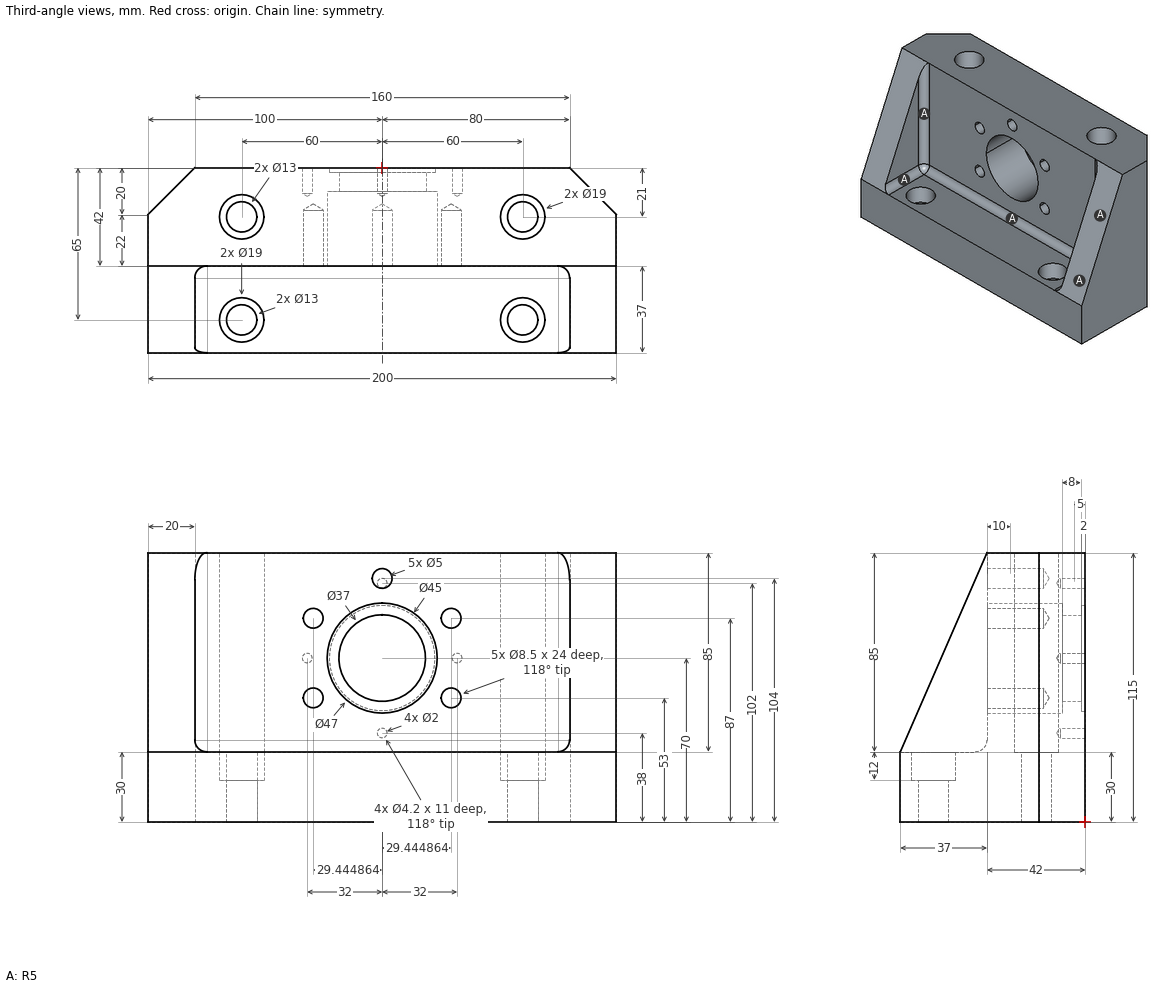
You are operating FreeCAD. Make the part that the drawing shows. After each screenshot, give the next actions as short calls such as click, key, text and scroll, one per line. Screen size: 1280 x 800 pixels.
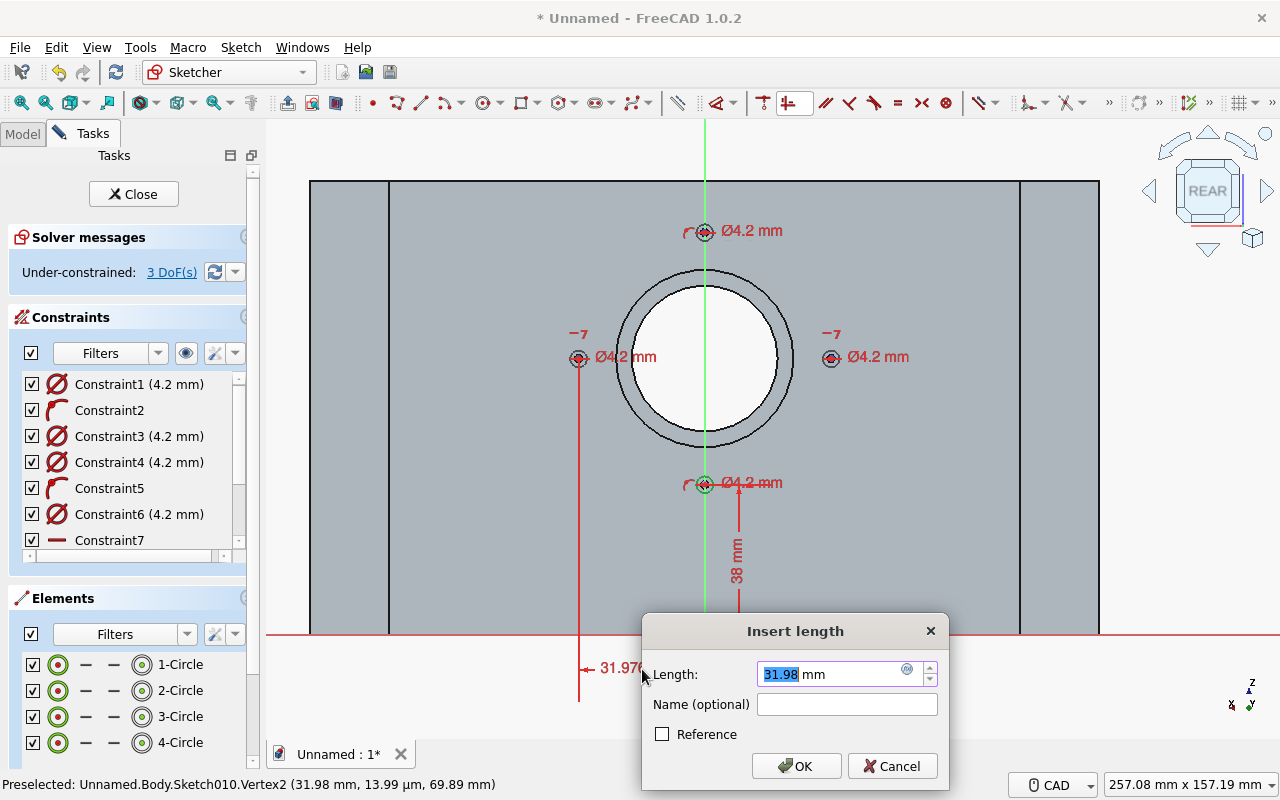
text(32)
key(Return)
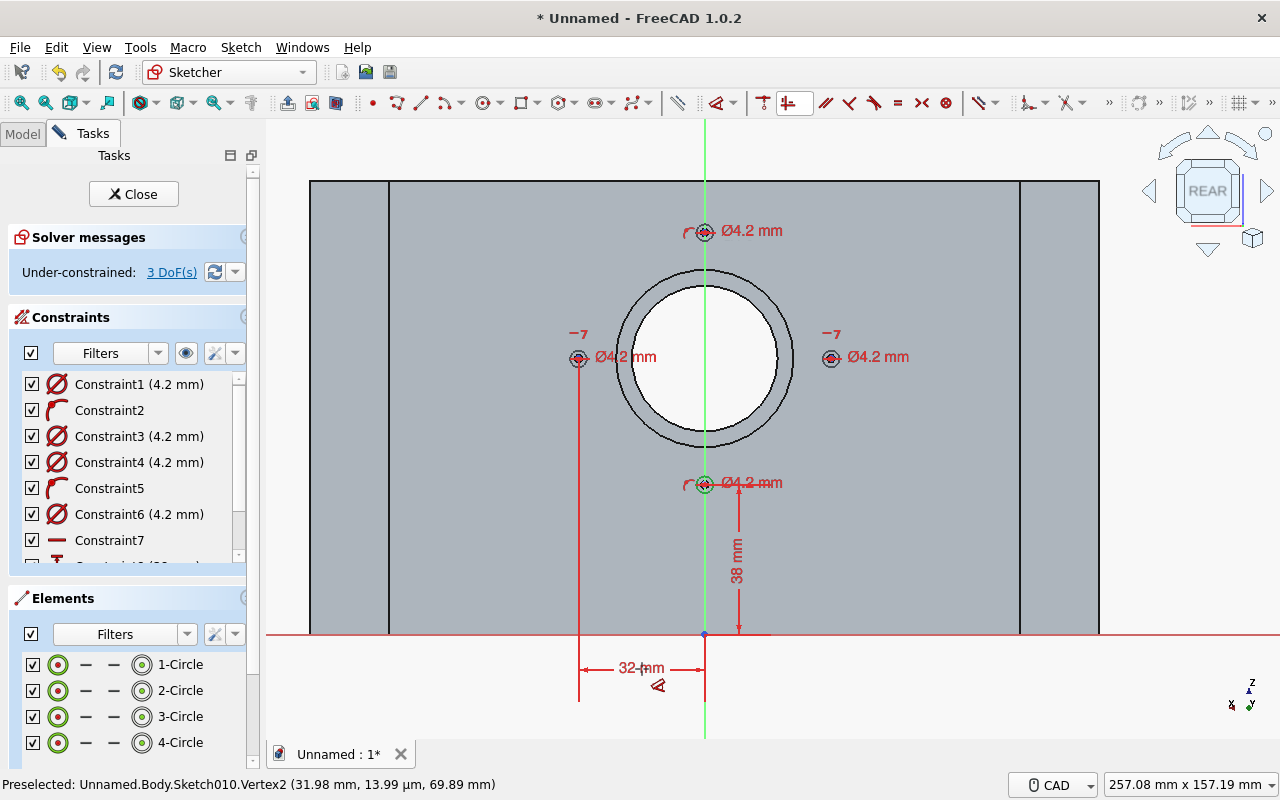
click(579, 359)
click(545, 497)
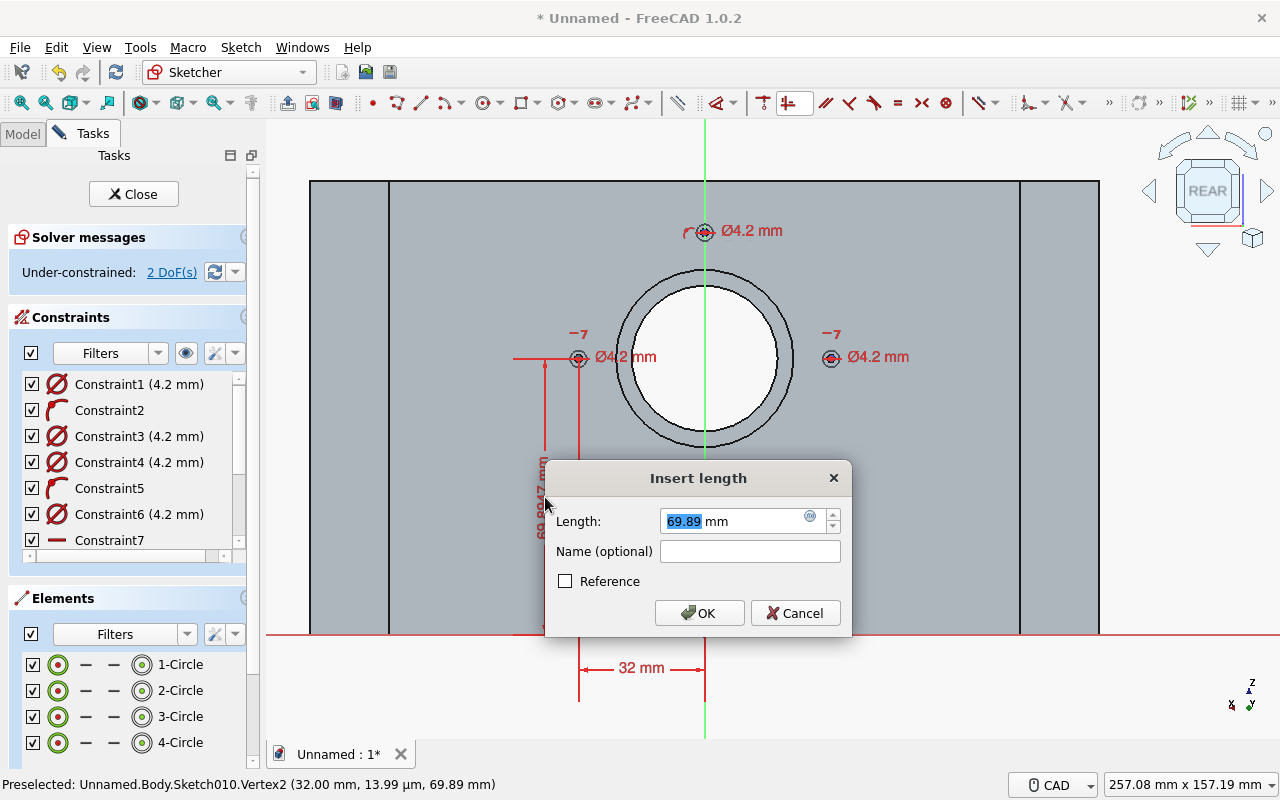
text(70)
key(Return)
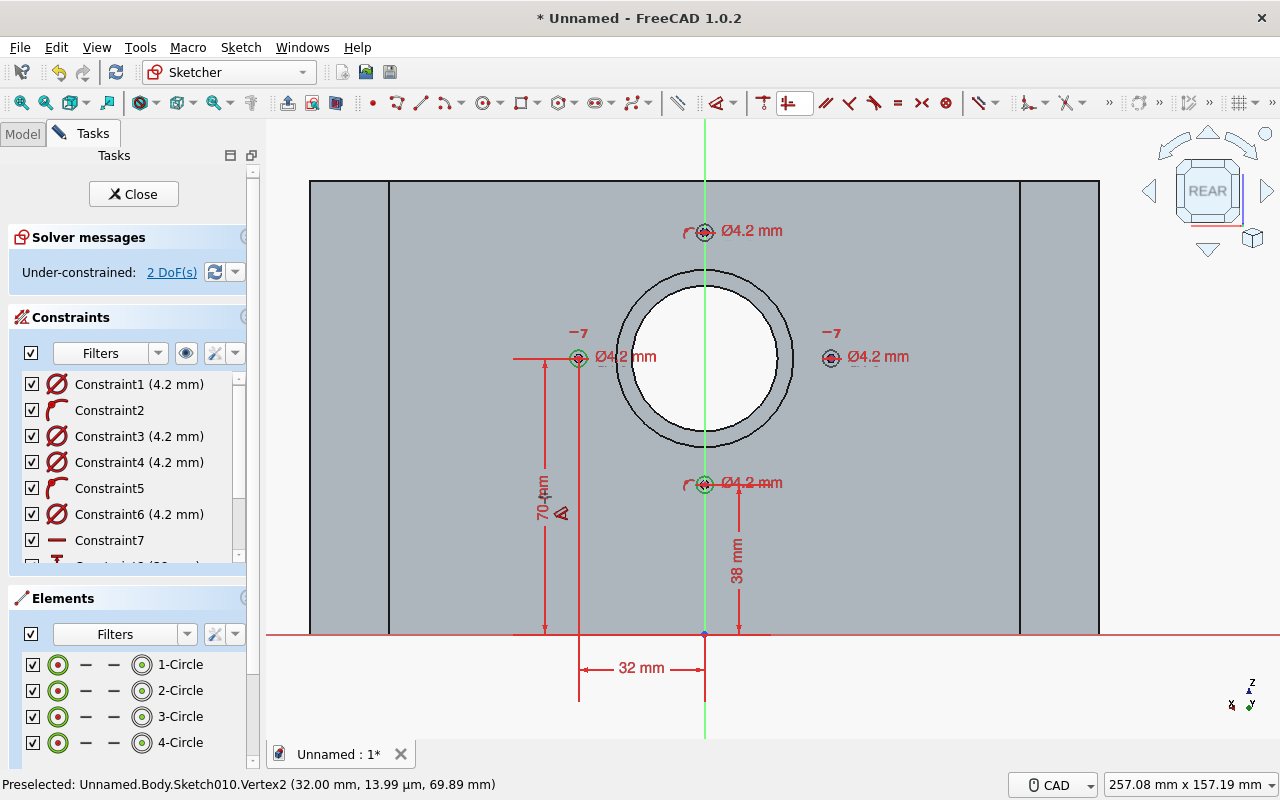
click(831, 359)
click(768, 669)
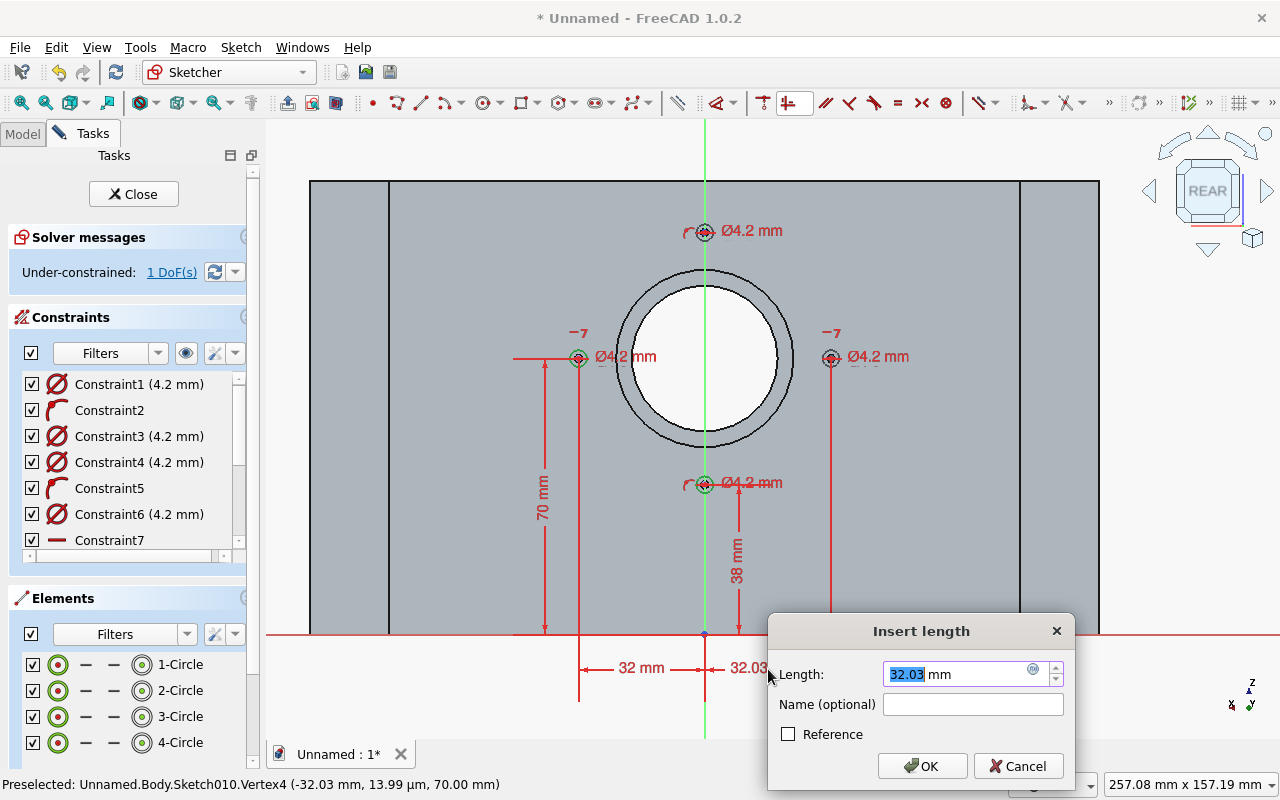
text(32)
key(Return)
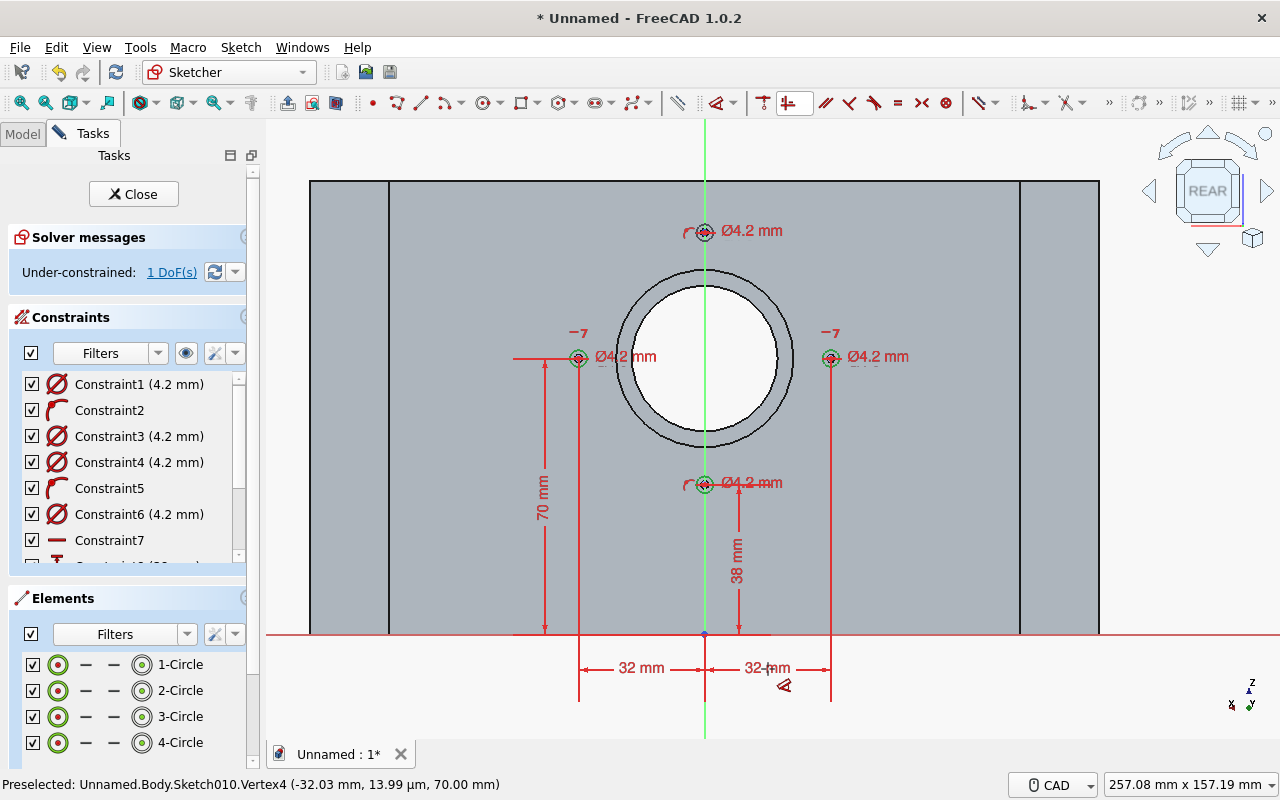
click(705, 233)
click(739, 434)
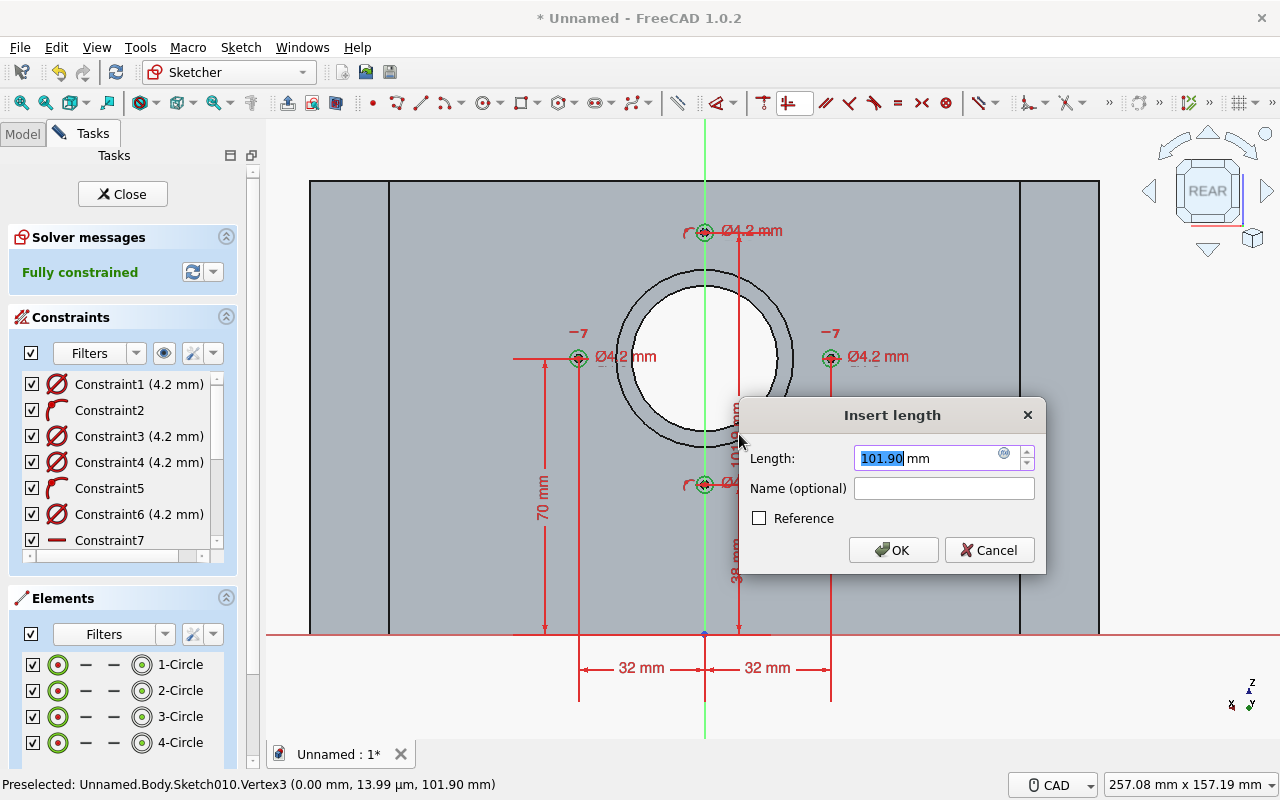
text(102)
key(Return)
key(Escape)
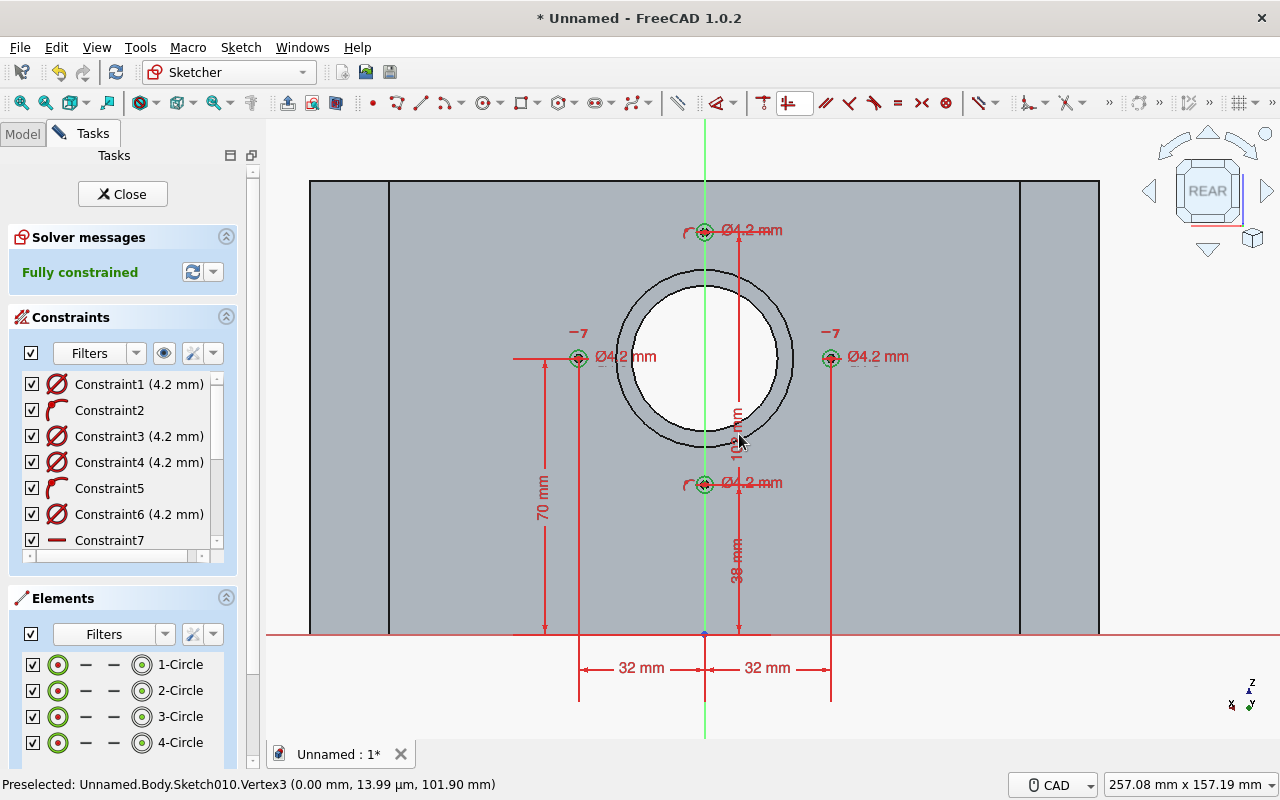
click(123, 194)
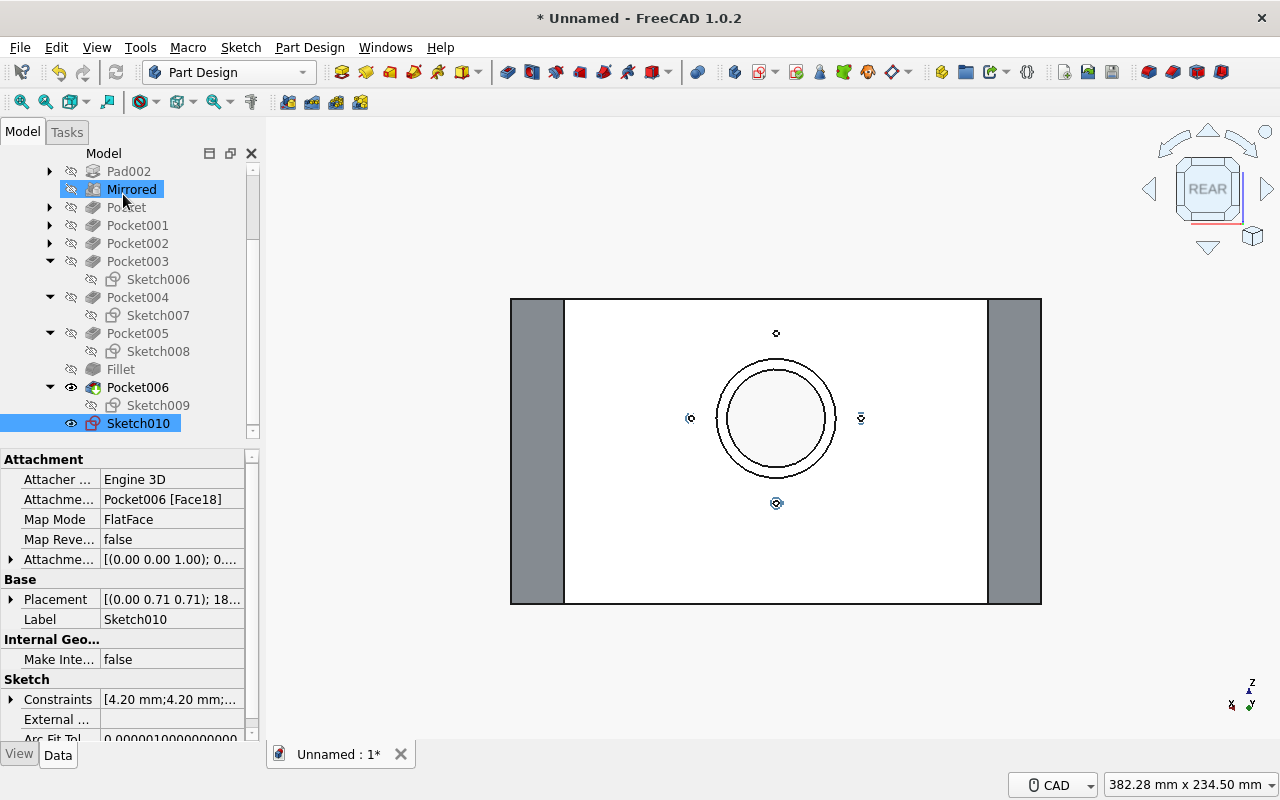
click(532, 72)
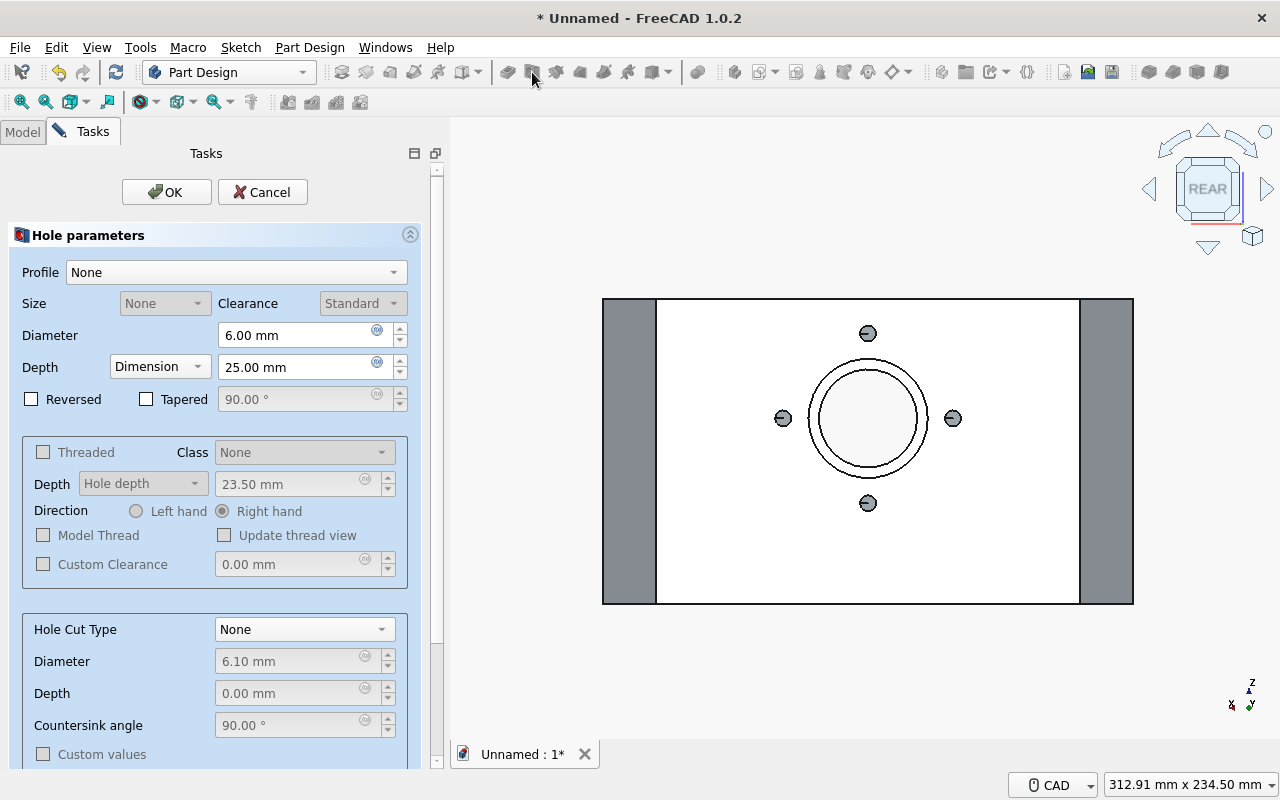
triple_click(305, 335)